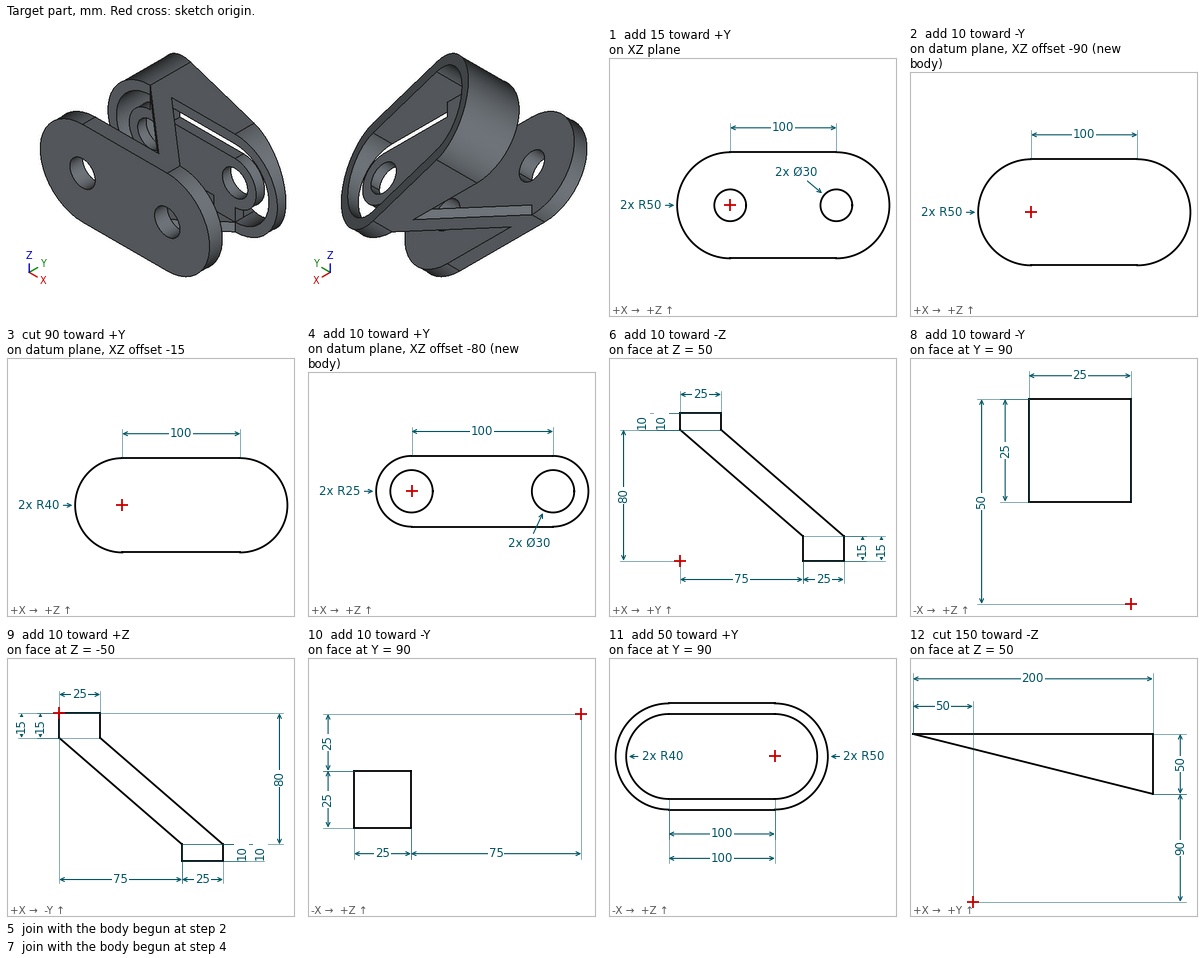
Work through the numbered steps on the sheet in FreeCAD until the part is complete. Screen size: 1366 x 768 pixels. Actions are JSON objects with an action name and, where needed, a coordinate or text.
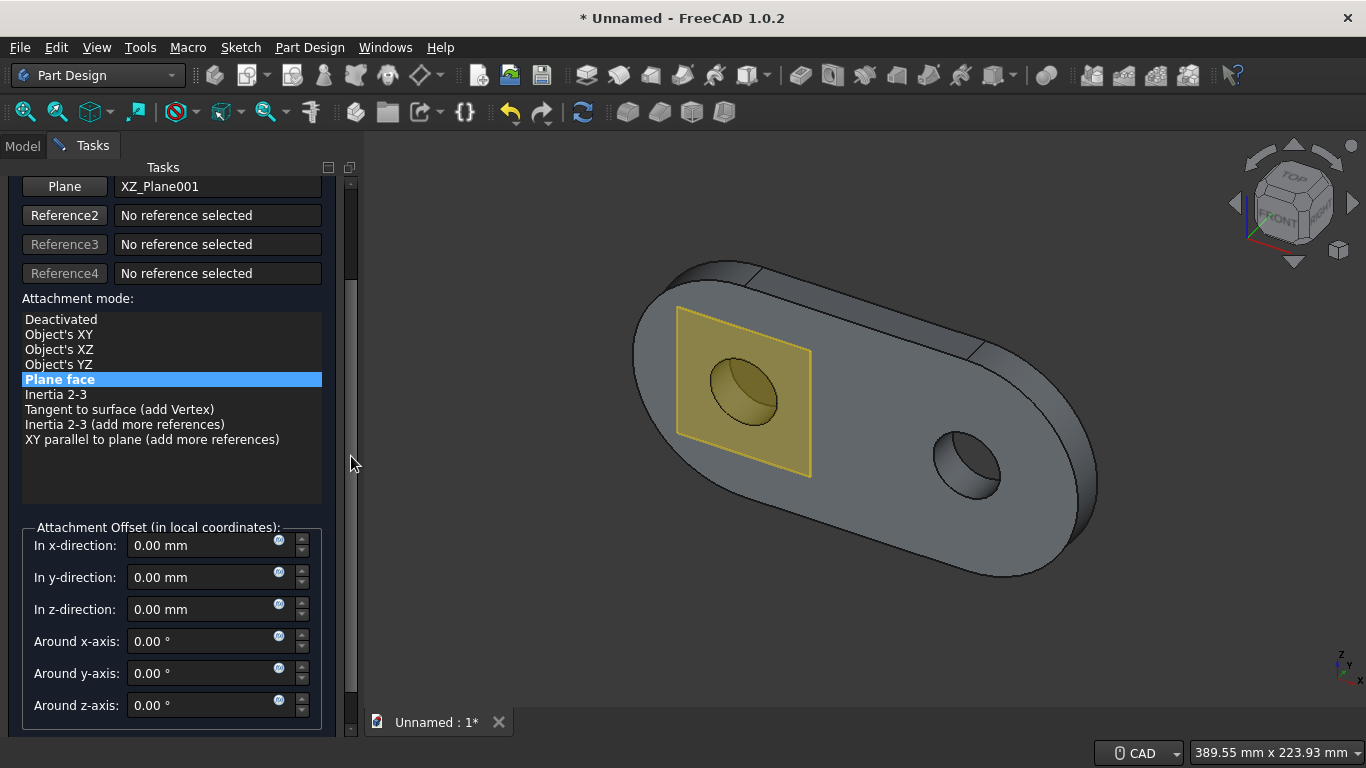
{"action": "triple_click", "coordinate": [210, 609]}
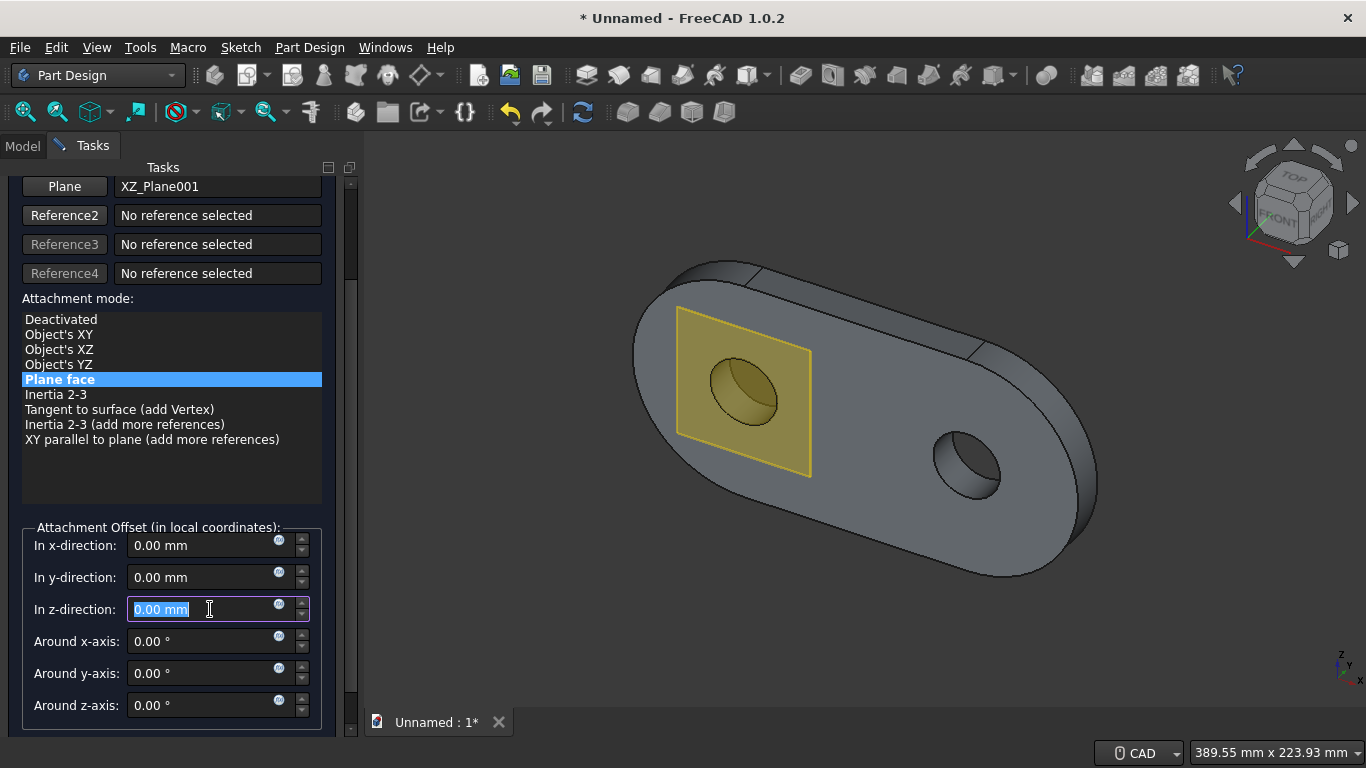
{"action": "type", "text": "-90"}
{"action": "key", "text": "Tab"}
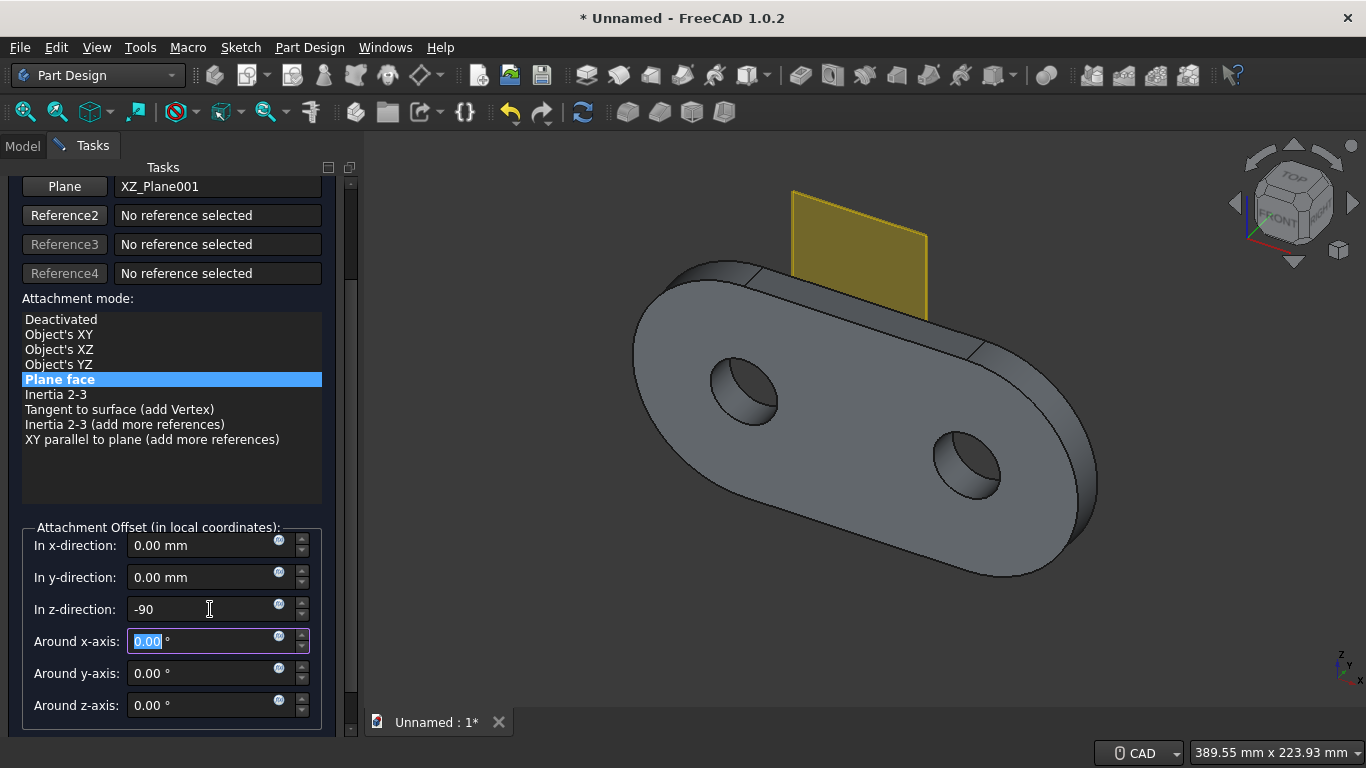
{"action": "scroll", "coordinate": [351, 456], "scroll_direction": "up", "scroll_amount": 3}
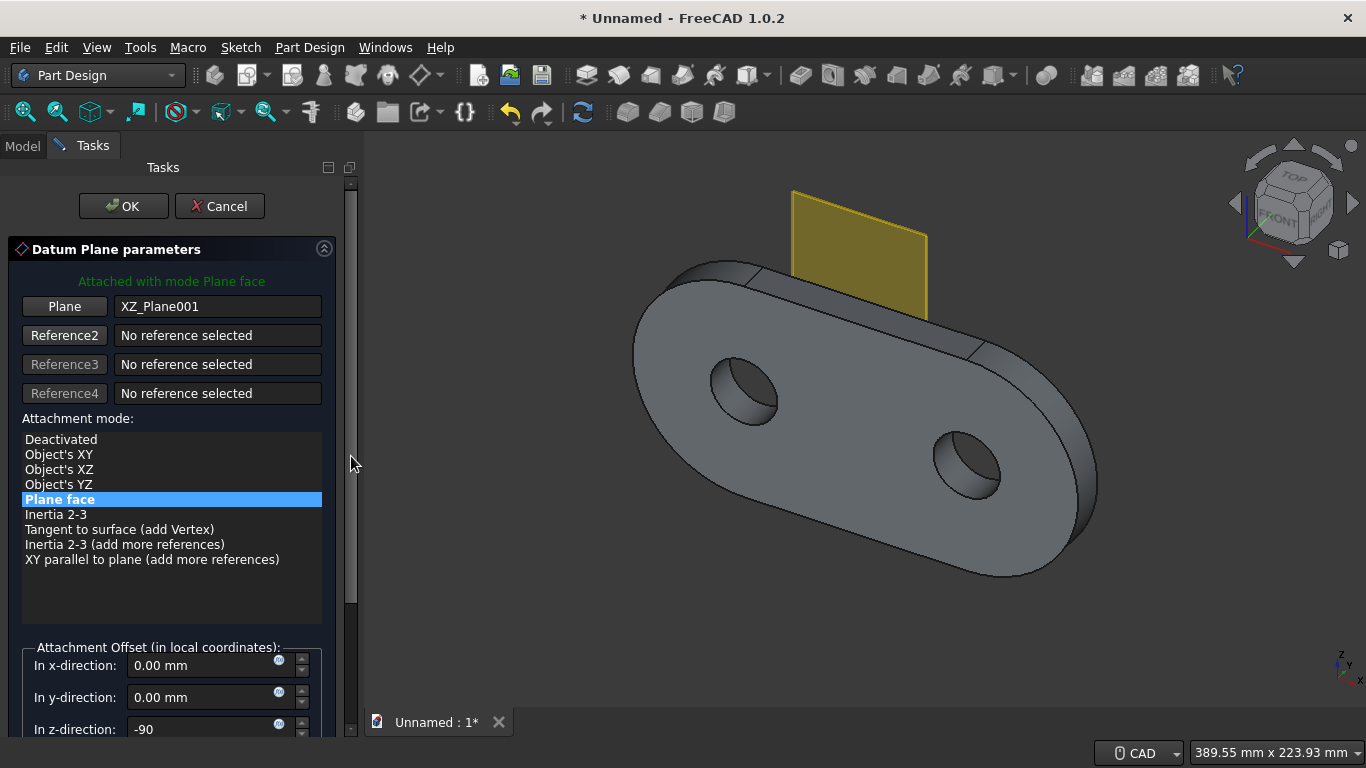
{"action": "left_click", "coordinate": [124, 206]}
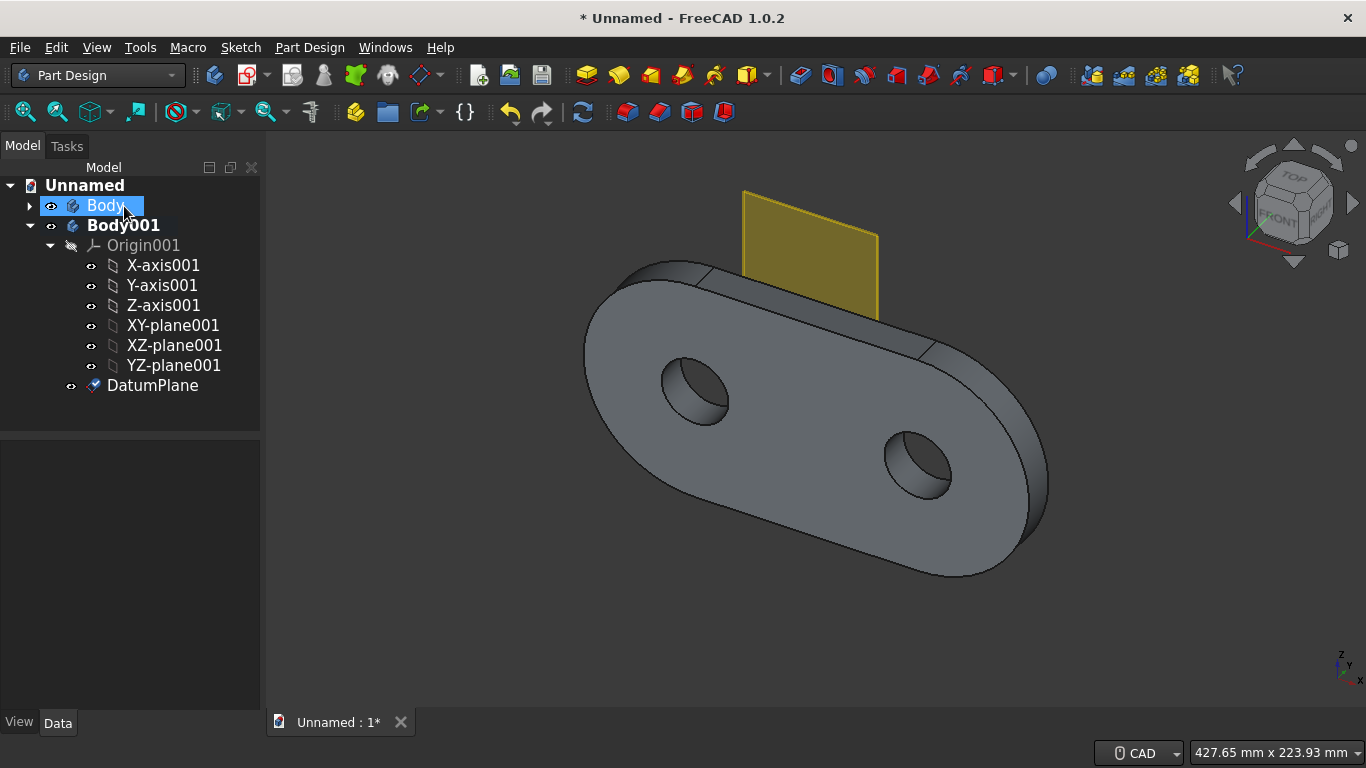
{"action": "left_click", "coordinate": [116, 386]}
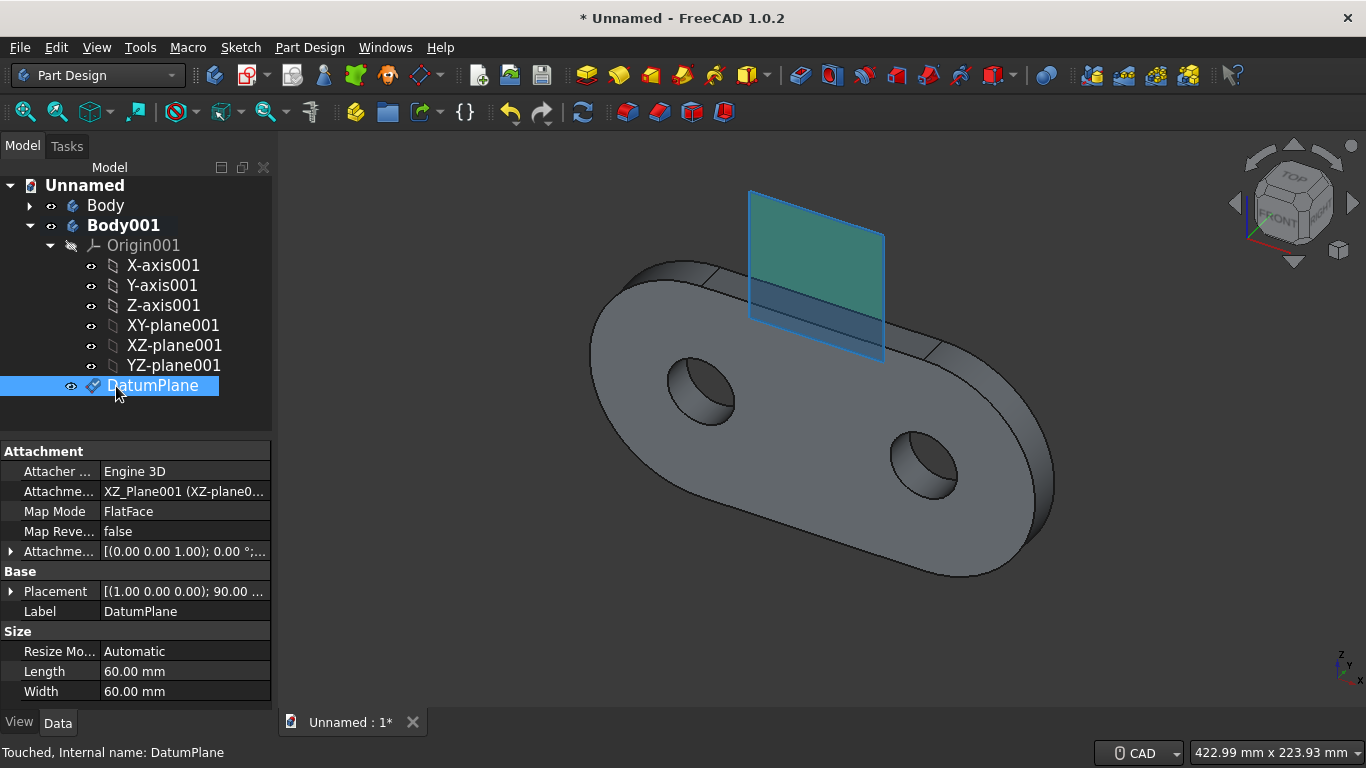
{"action": "left_click", "coordinate": [248, 76]}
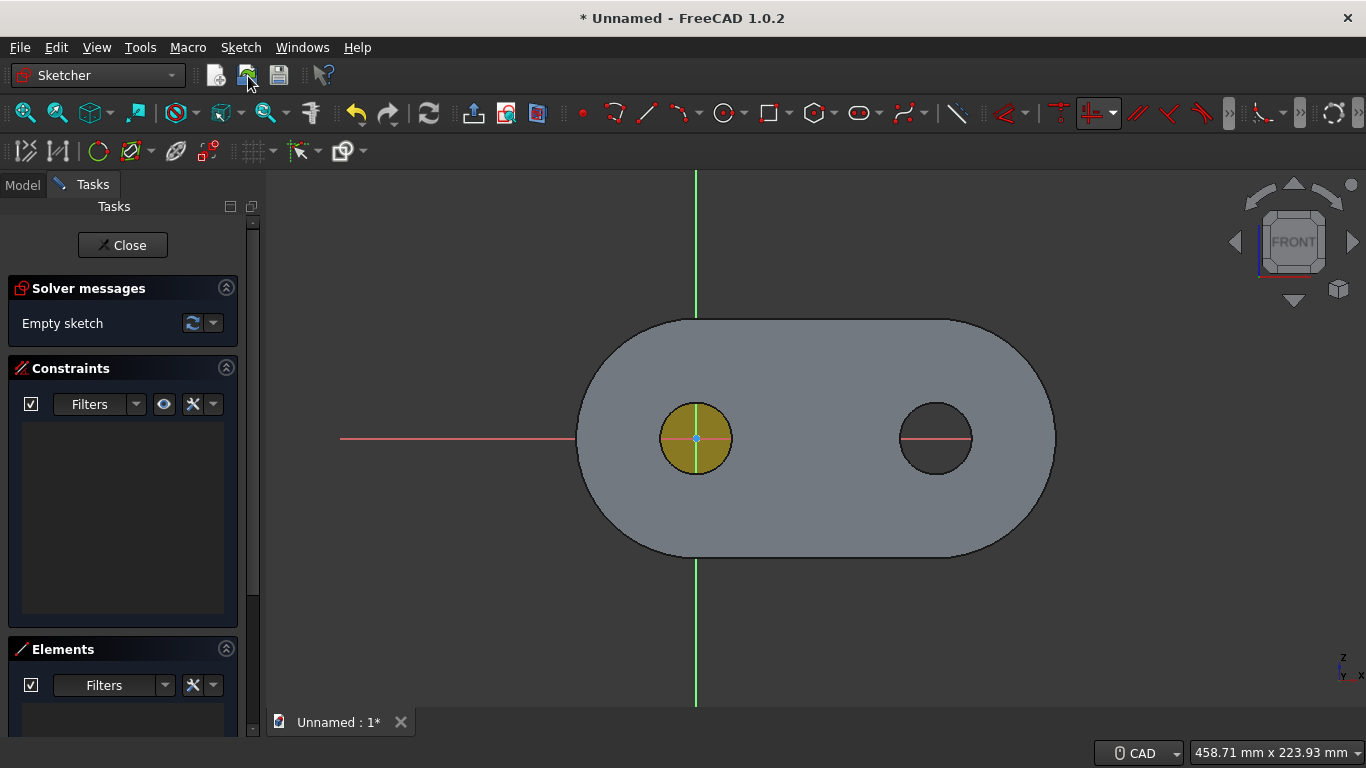
{"action": "left_click", "coordinate": [860, 114]}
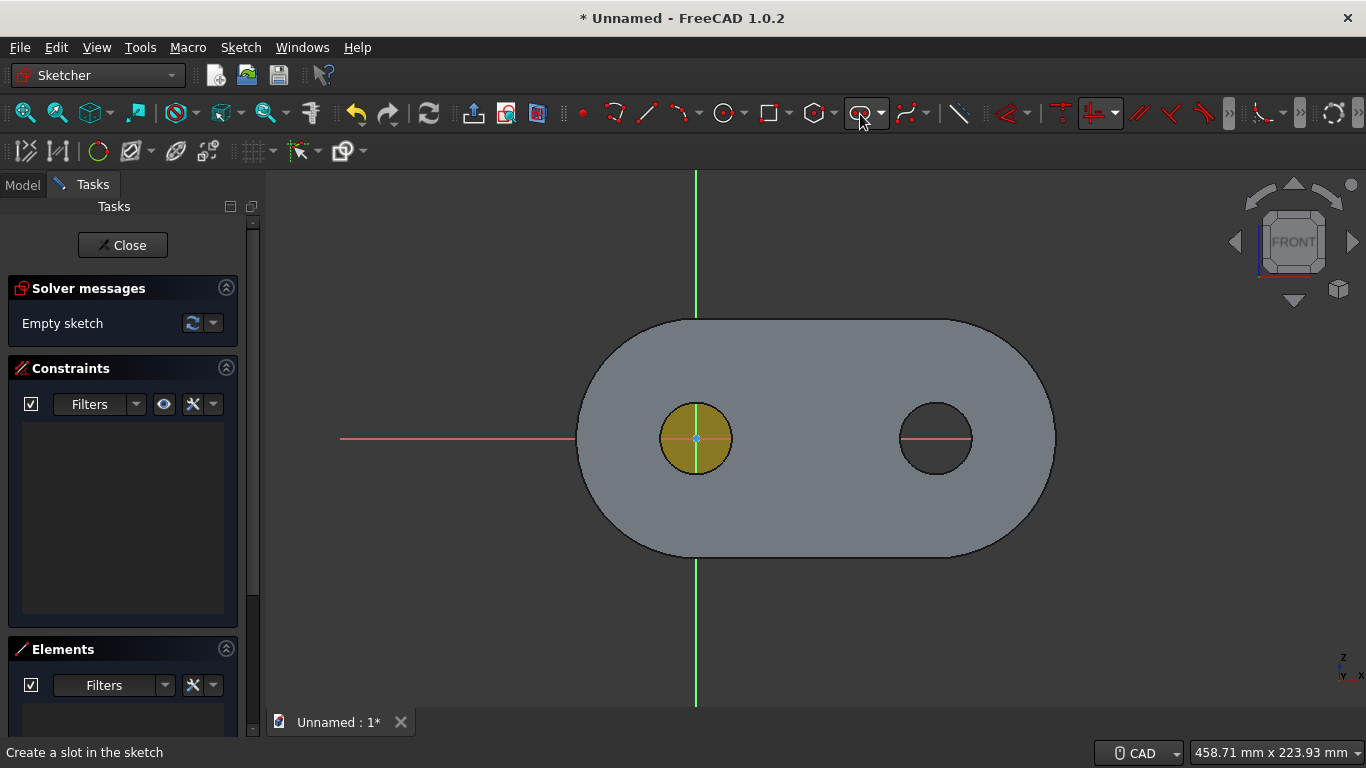
{"action": "left_click", "coordinate": [696, 439]}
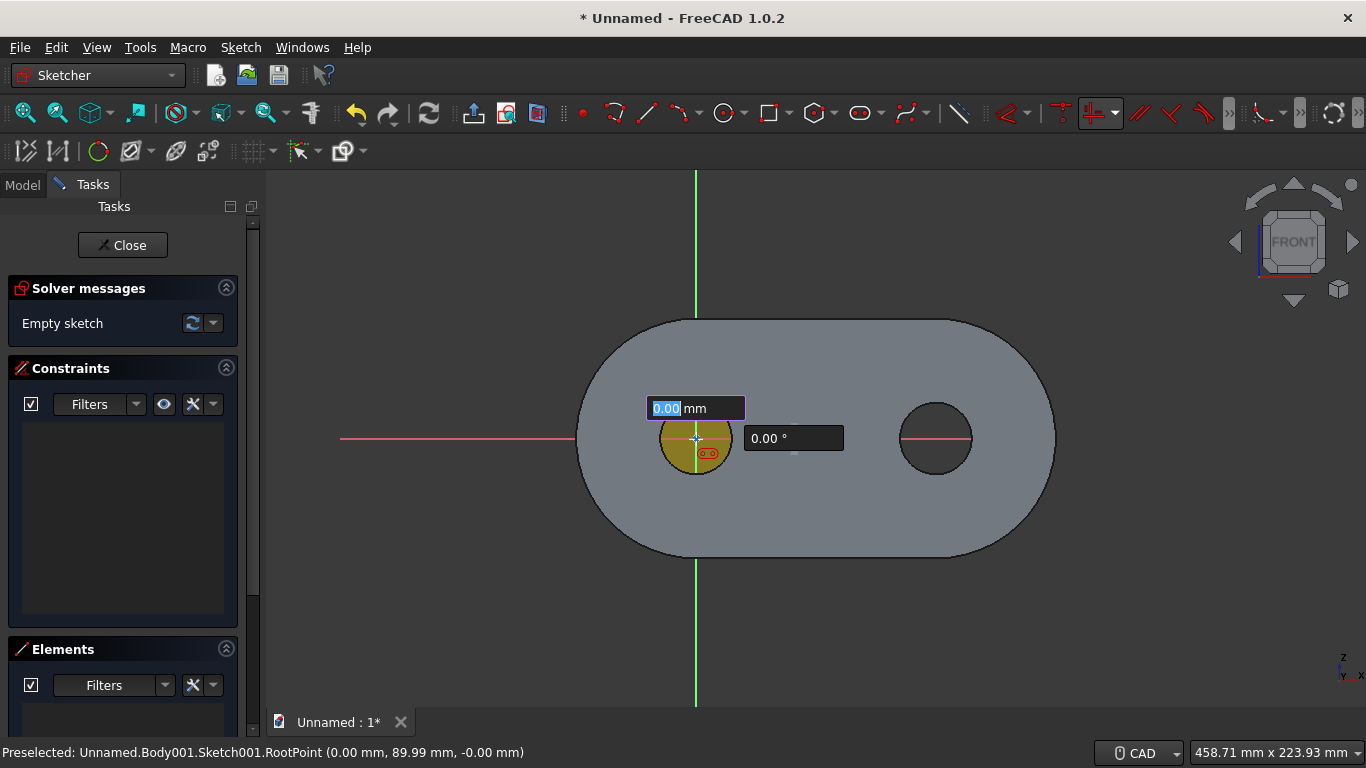
{"action": "left_click", "coordinate": [936, 430]}